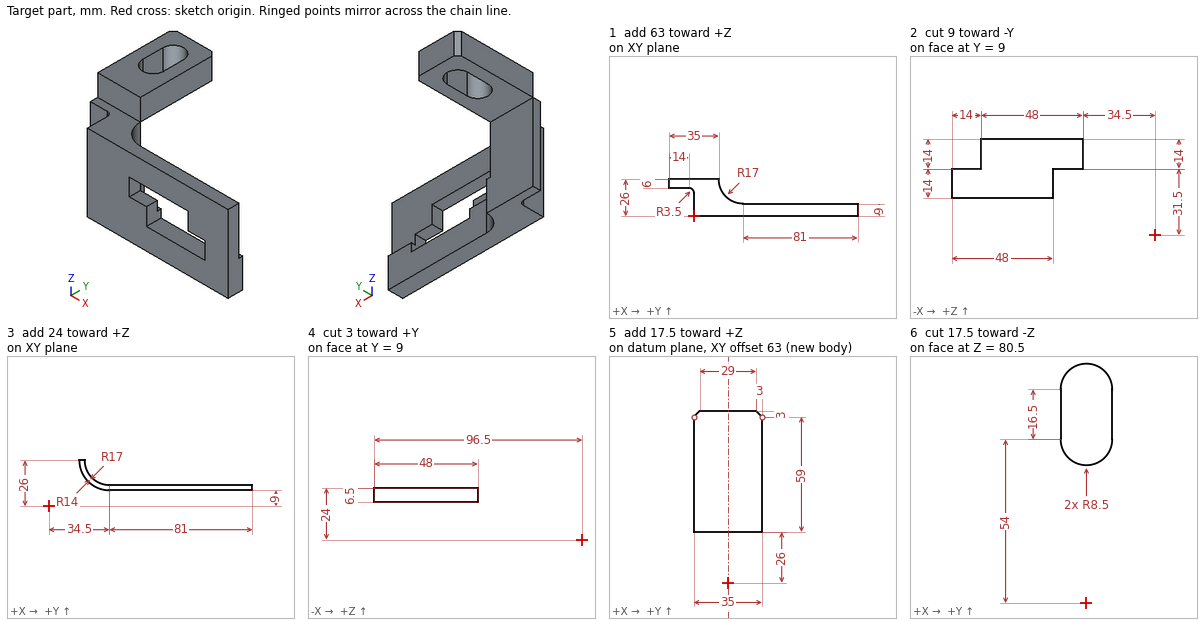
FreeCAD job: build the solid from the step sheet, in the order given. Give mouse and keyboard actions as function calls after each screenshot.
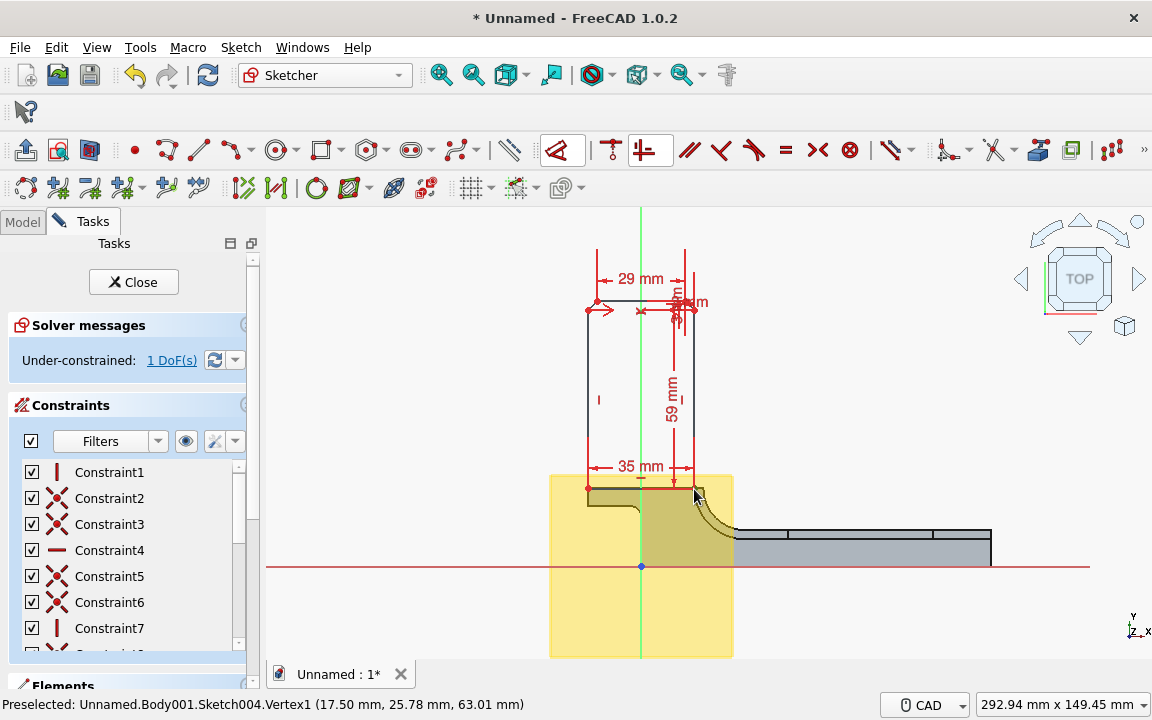
key(i)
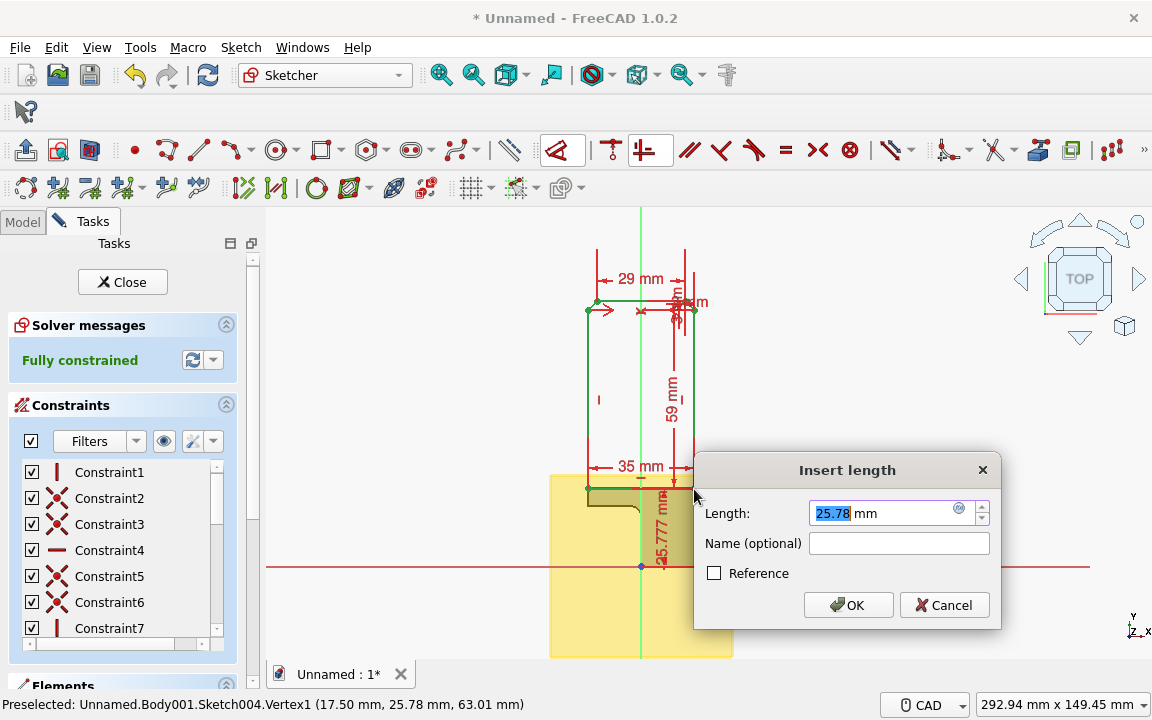
text(26)
key(Return)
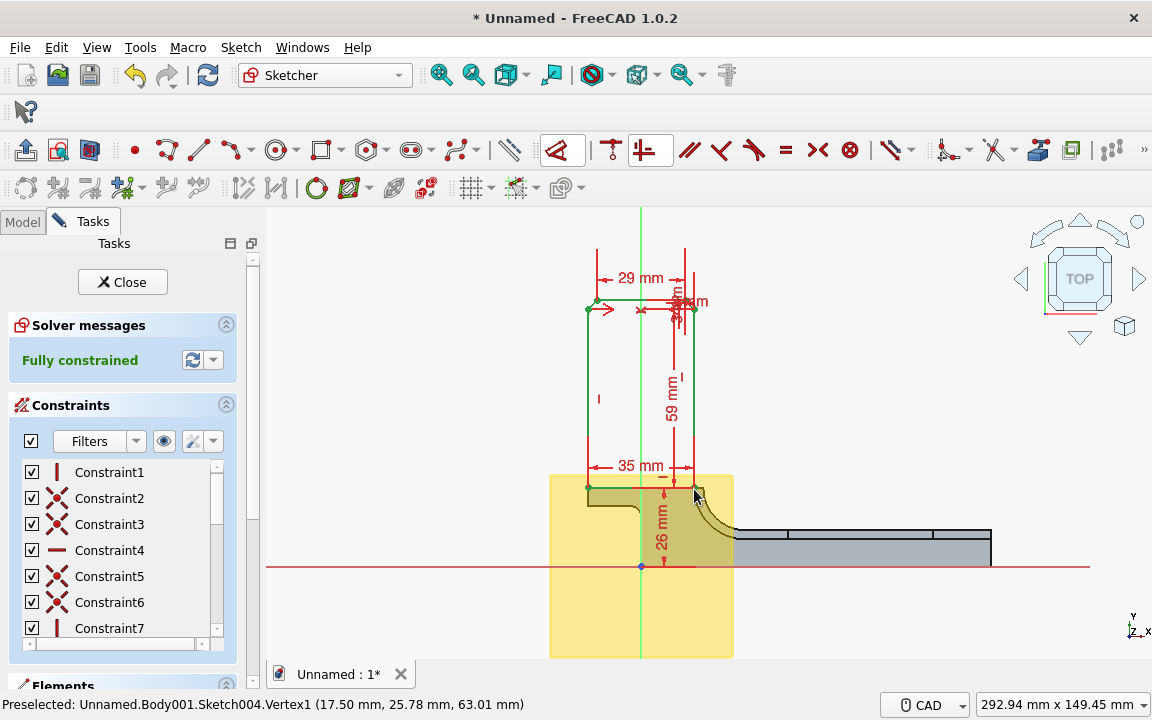
click(123, 282)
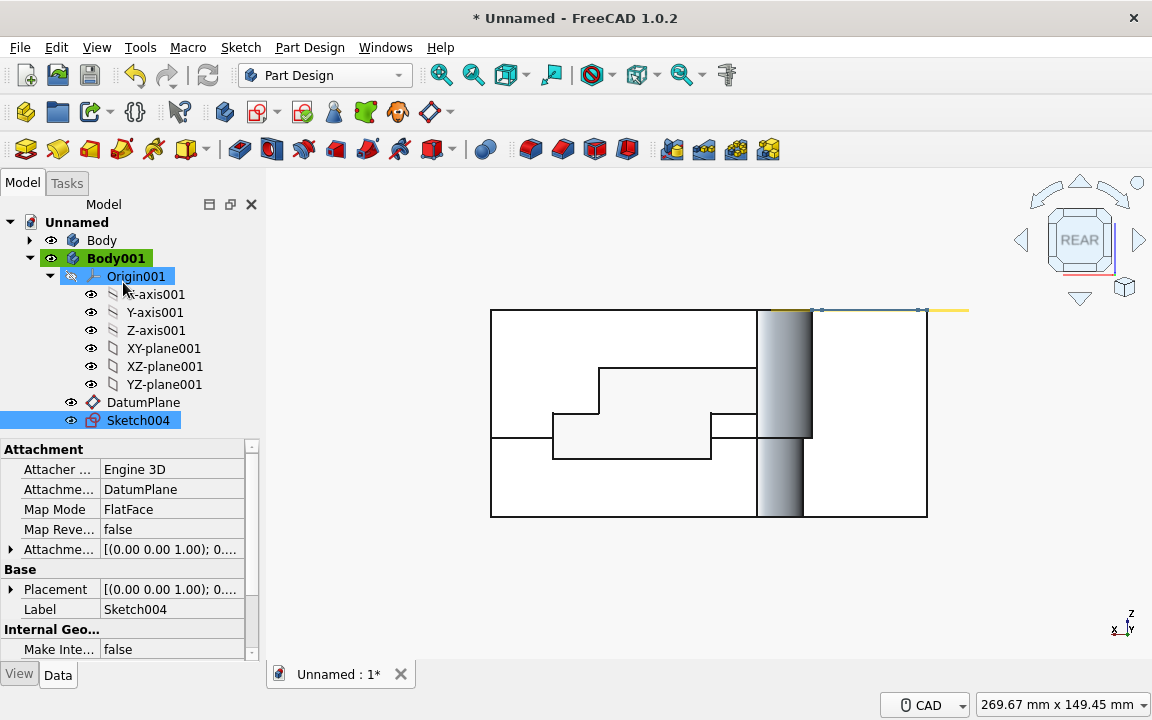
click(26, 150)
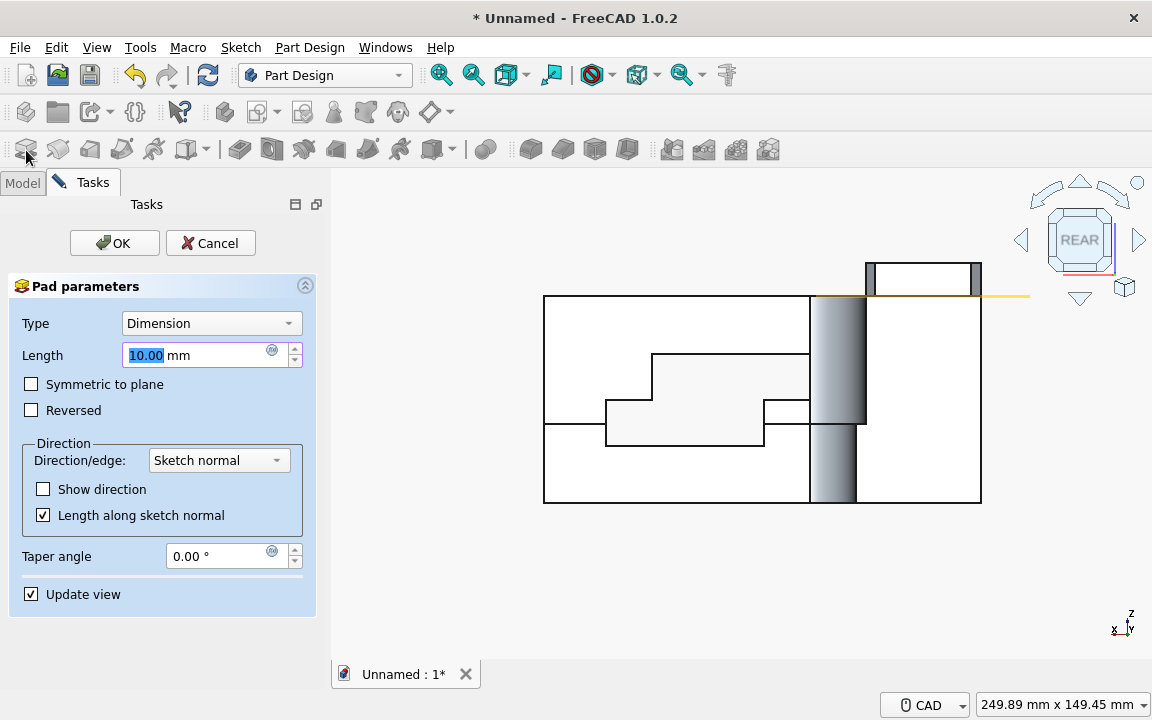
text(17.5)
key(Tab)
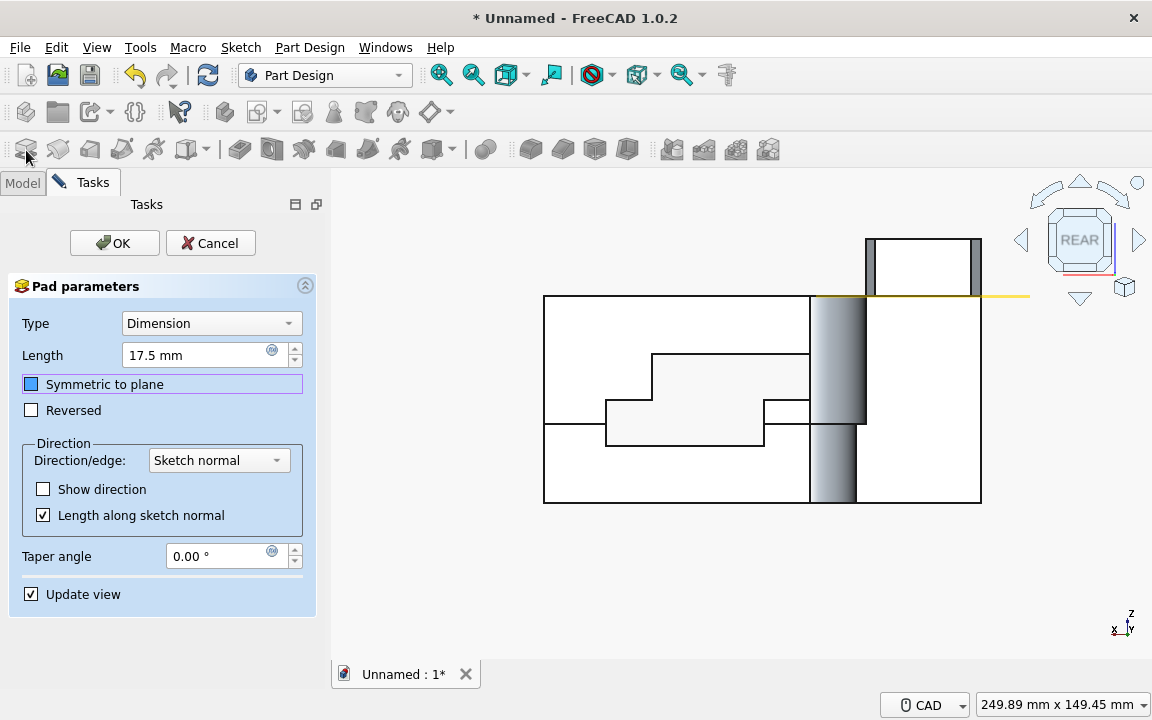
click(115, 243)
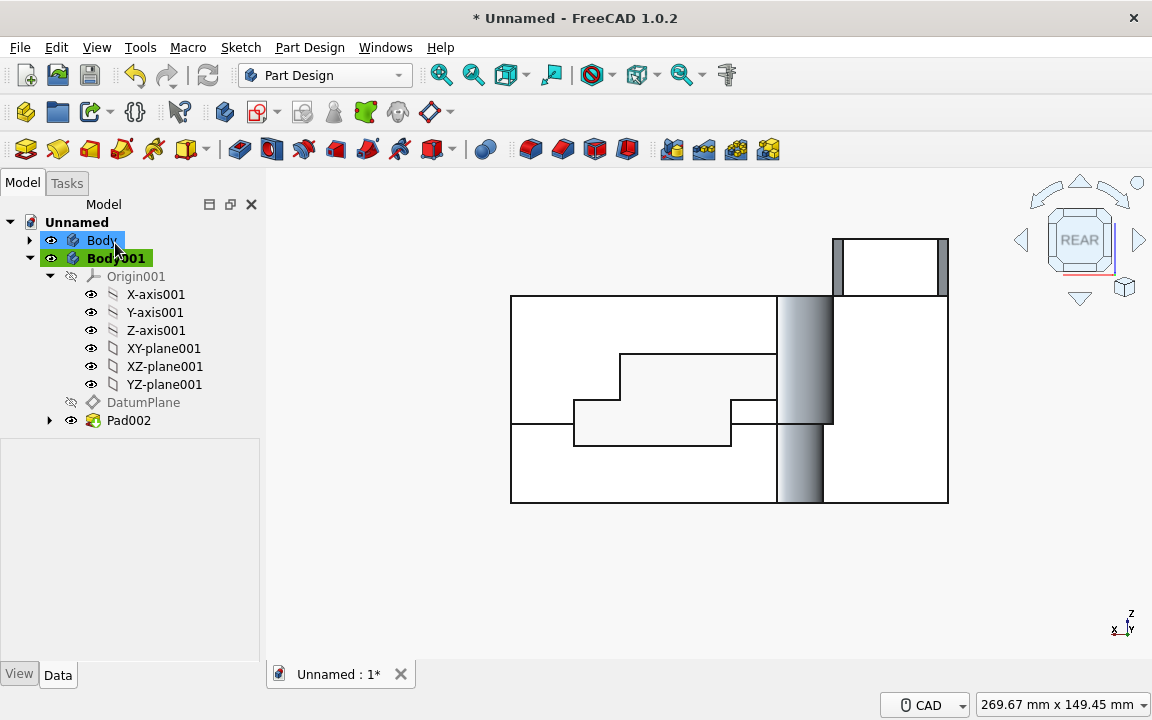
key(v)
key(f)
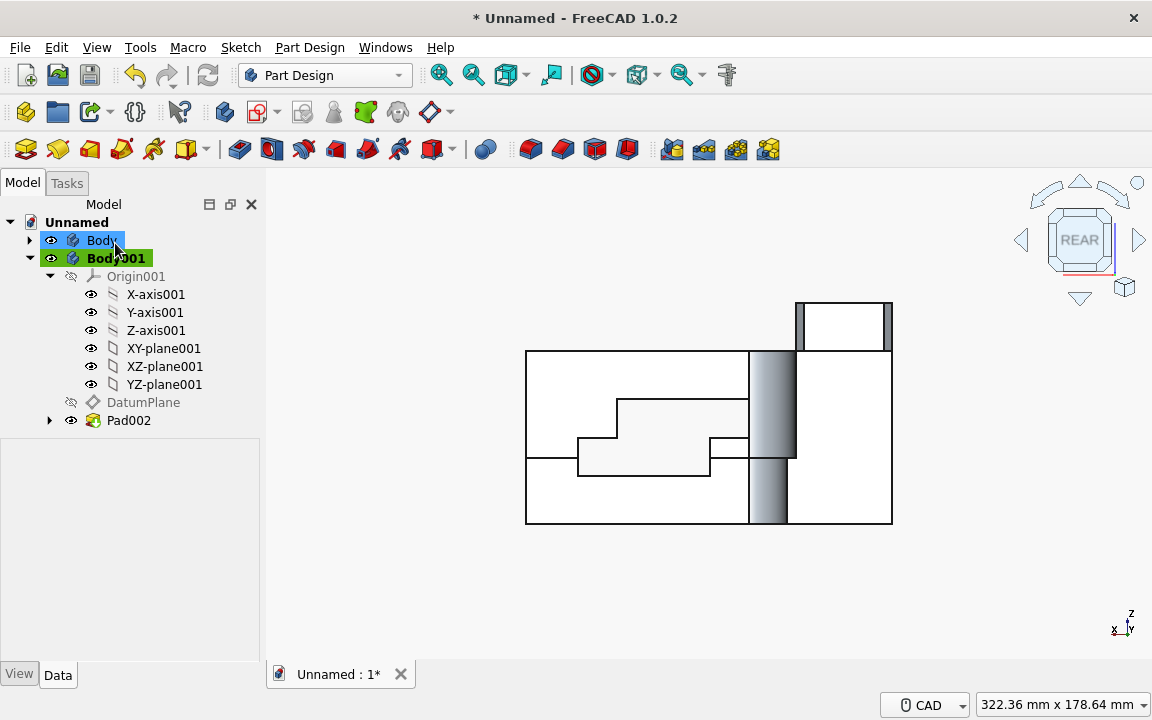
key(0)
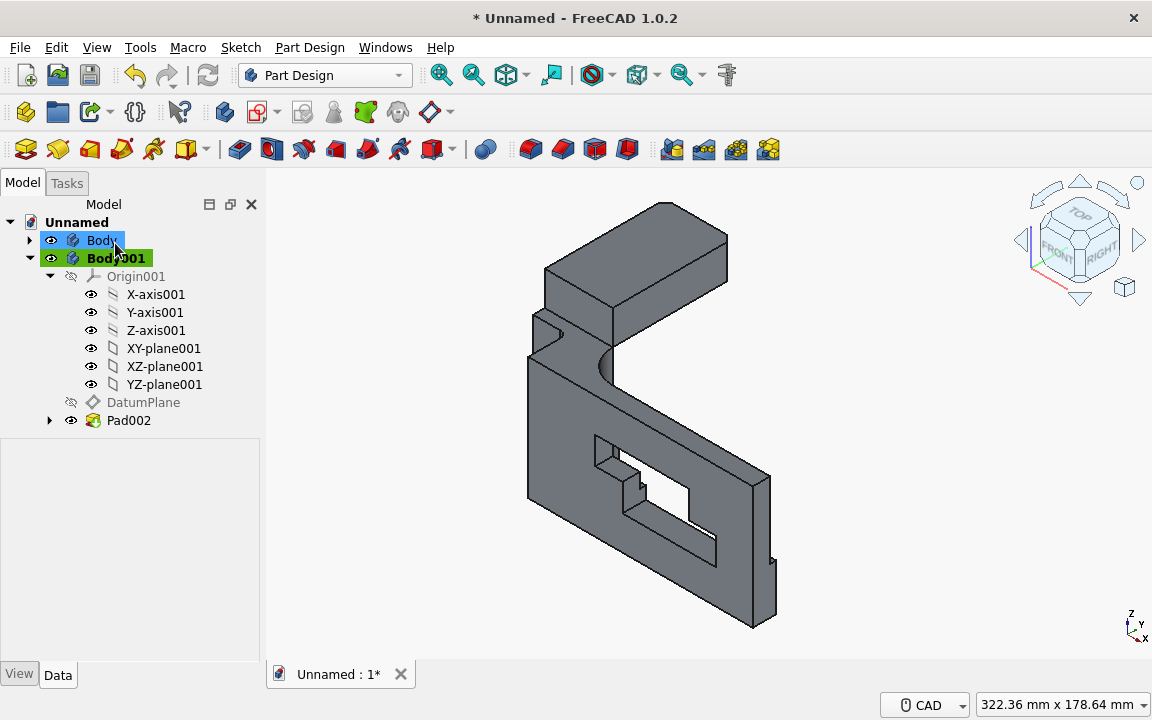
key(v)
key(f)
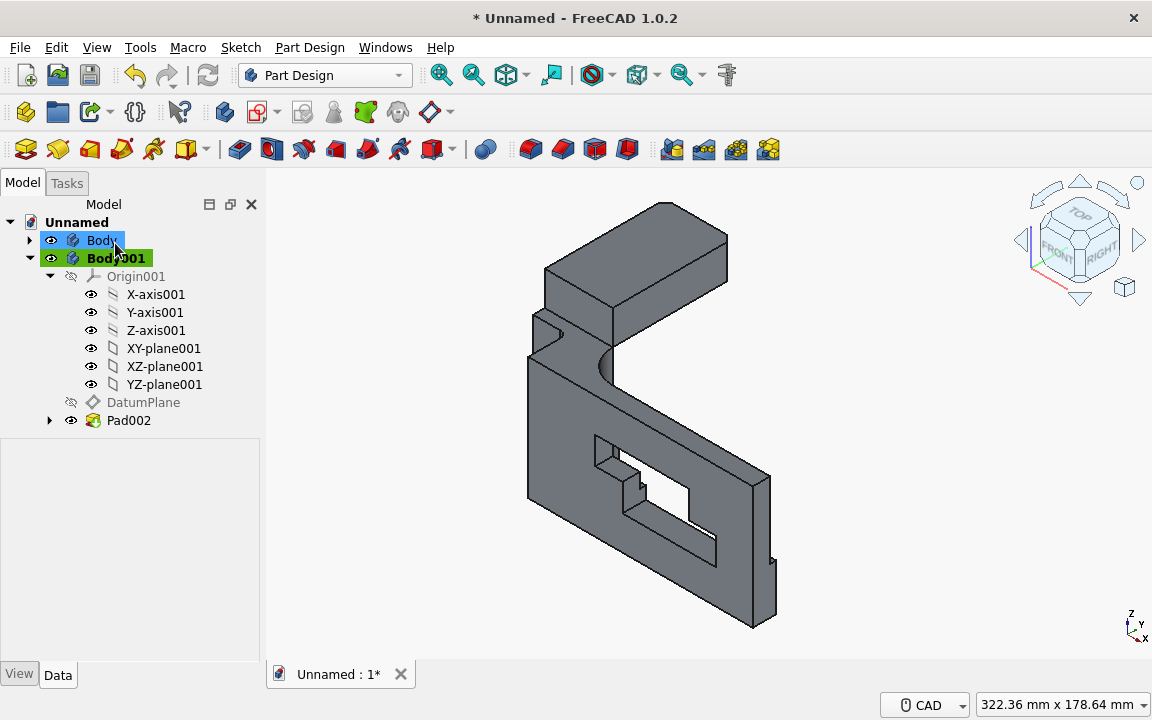
click(656, 243)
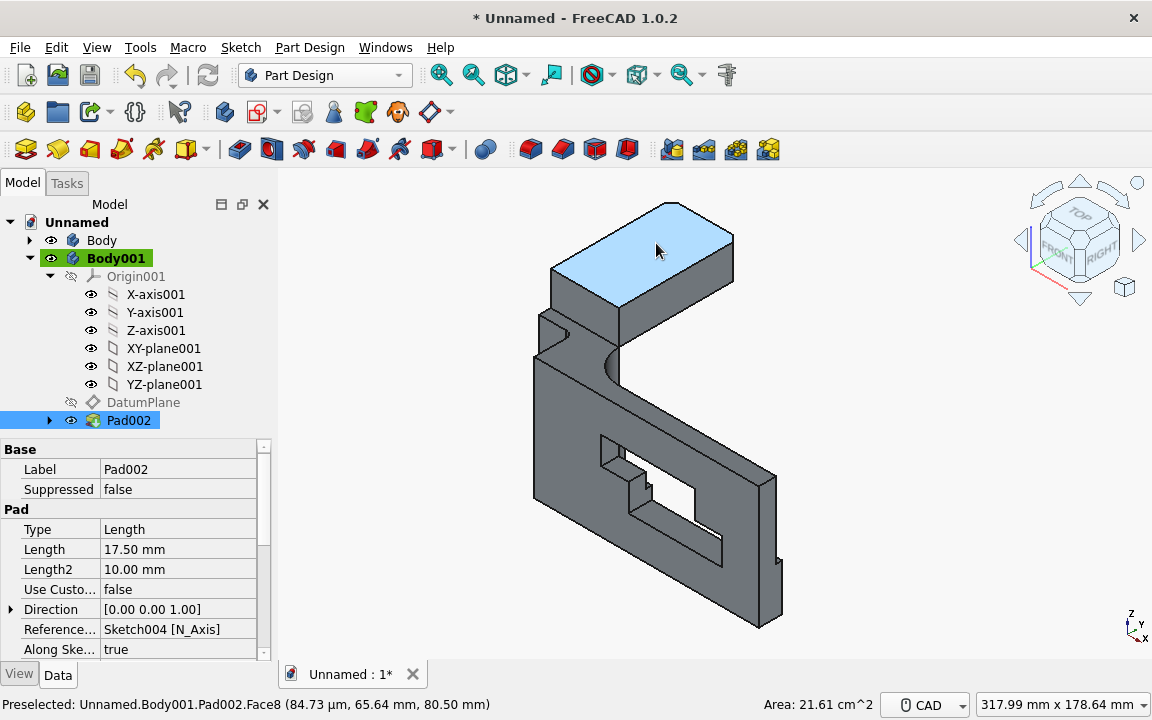
click(258, 112)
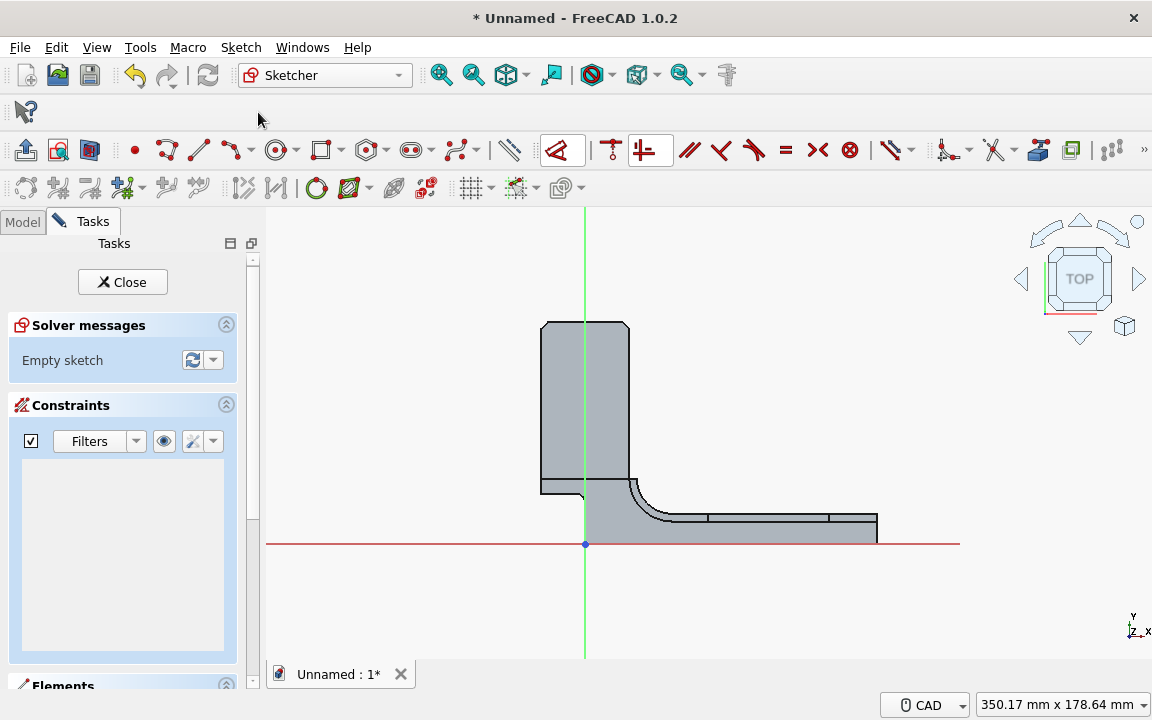
scroll(472, 468, up, 2)